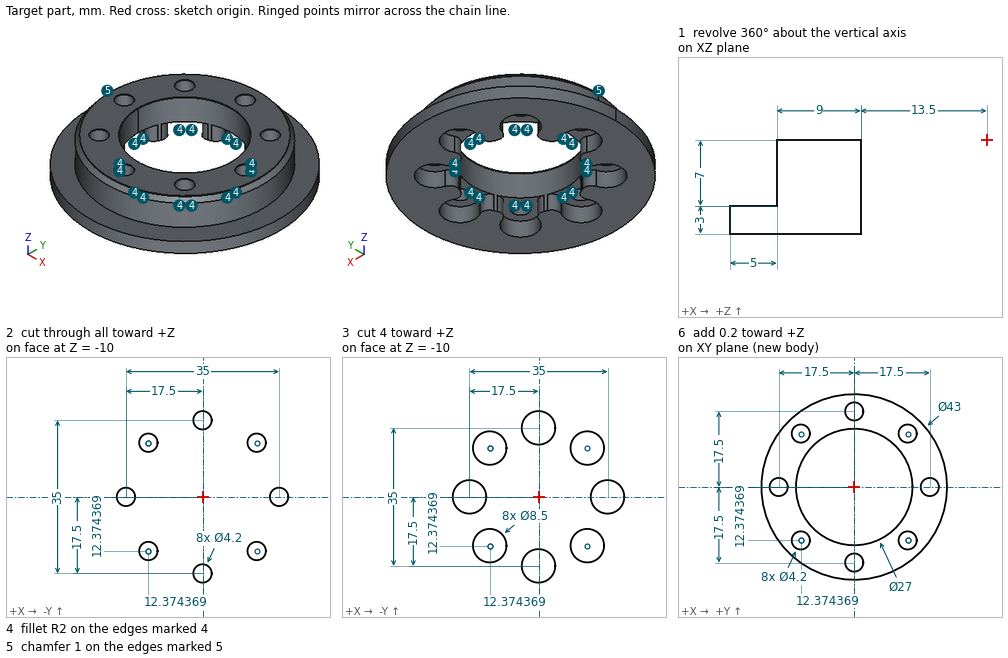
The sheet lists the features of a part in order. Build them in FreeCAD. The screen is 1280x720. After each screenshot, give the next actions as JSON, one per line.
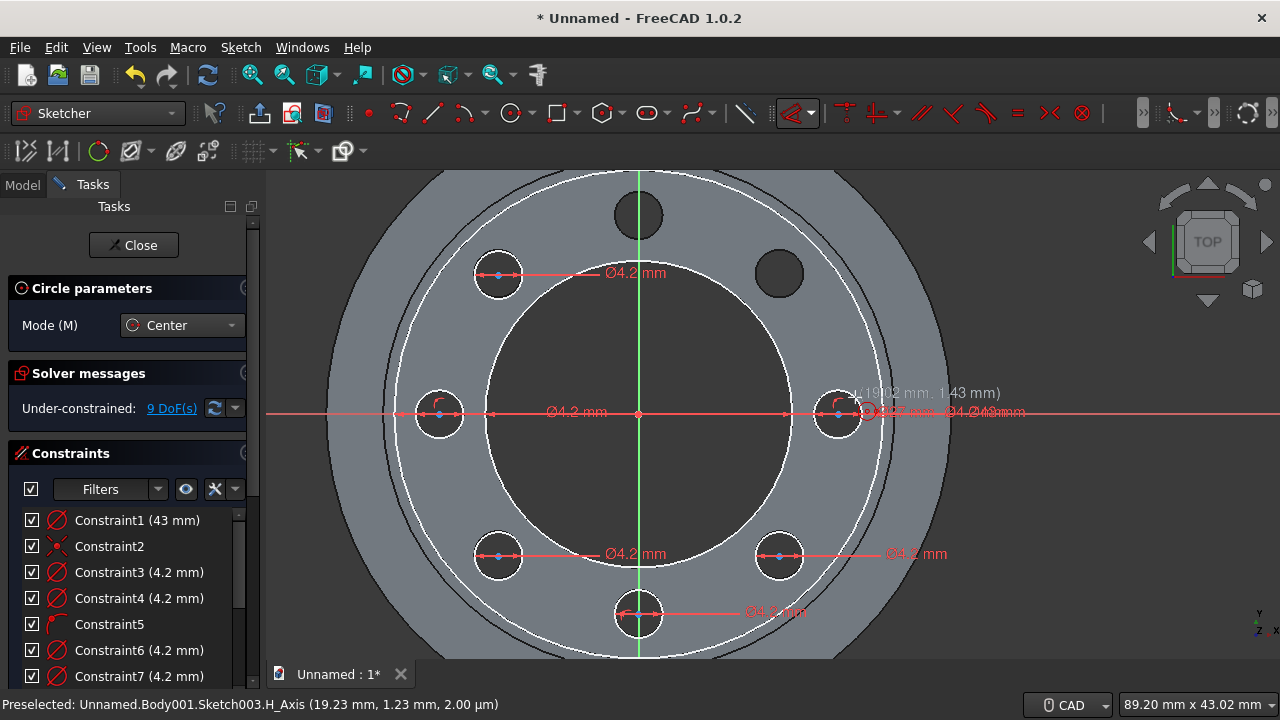
{"action": "left_click", "coordinate": [639, 215]}
{"action": "mouse_move", "coordinate": [656, 198]}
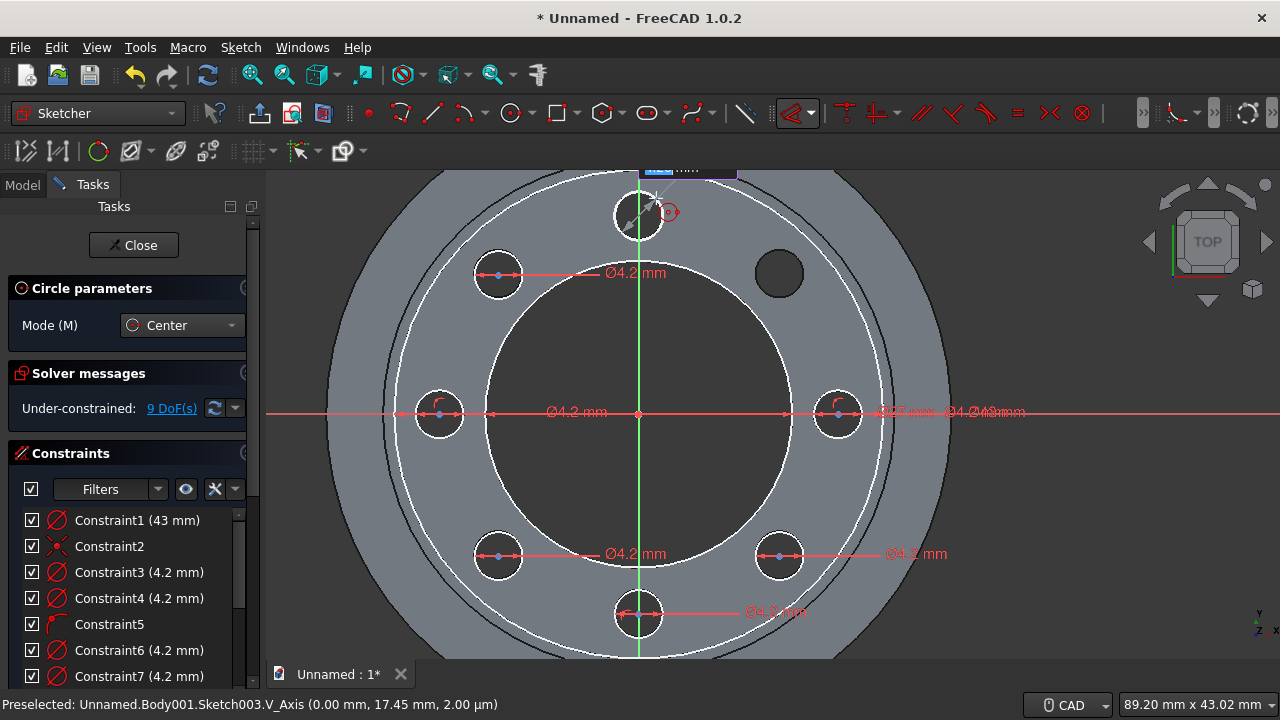
{"action": "type", "text": "4.2"}
{"action": "key", "text": "Return"}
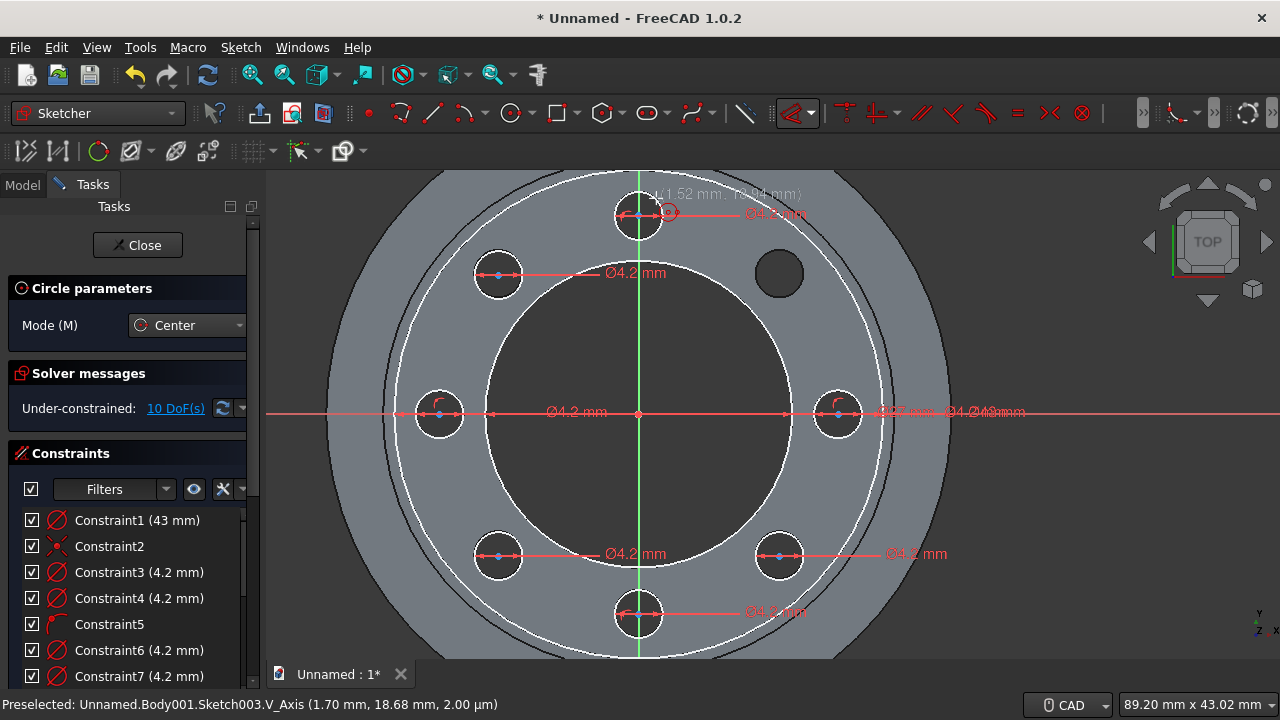
{"action": "left_click", "coordinate": [779, 274]}
{"action": "mouse_move", "coordinate": [796, 257]}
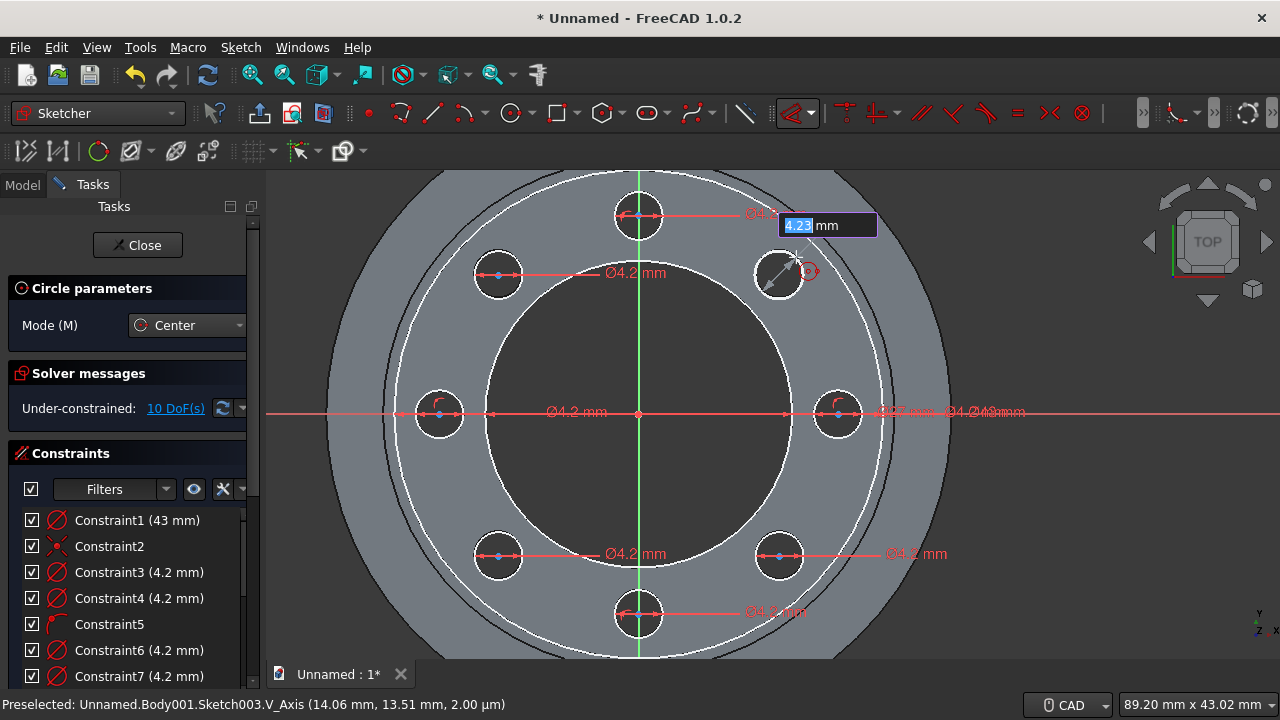
{"action": "type", "text": "4.2"}
{"action": "key", "text": "Return"}
{"action": "key", "text": "Escape"}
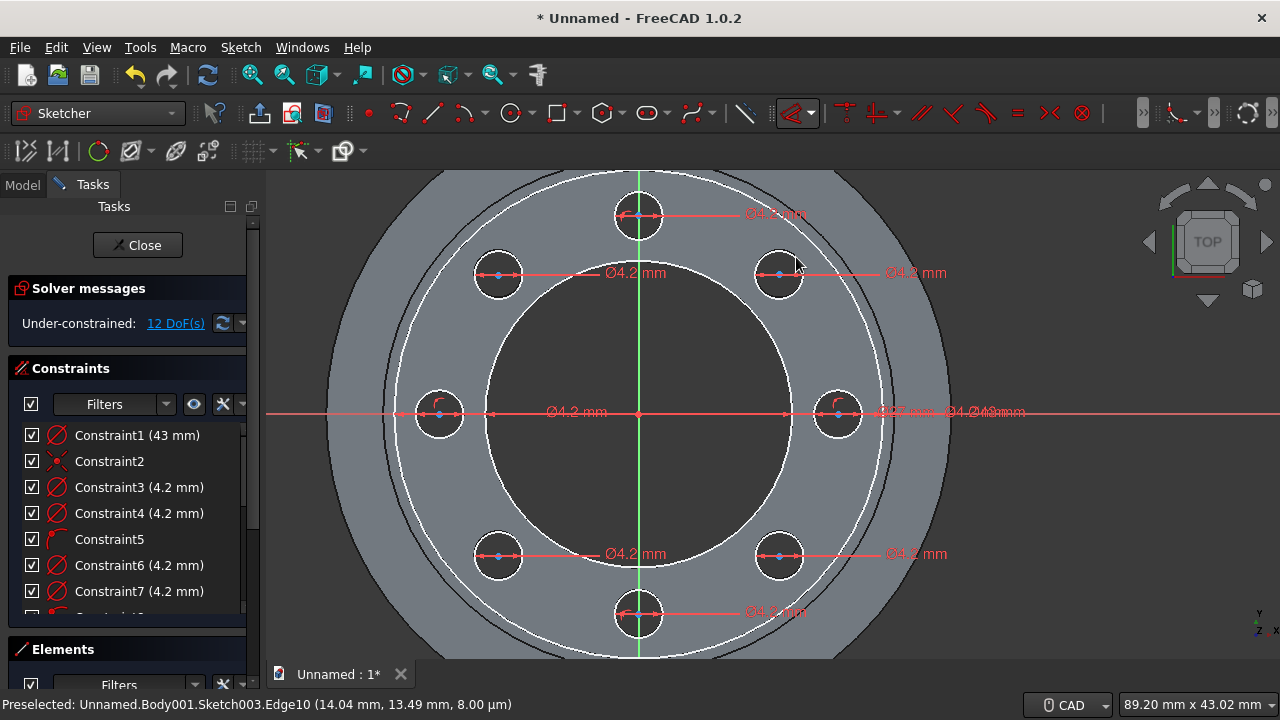
{"action": "left_click", "coordinate": [499, 556]}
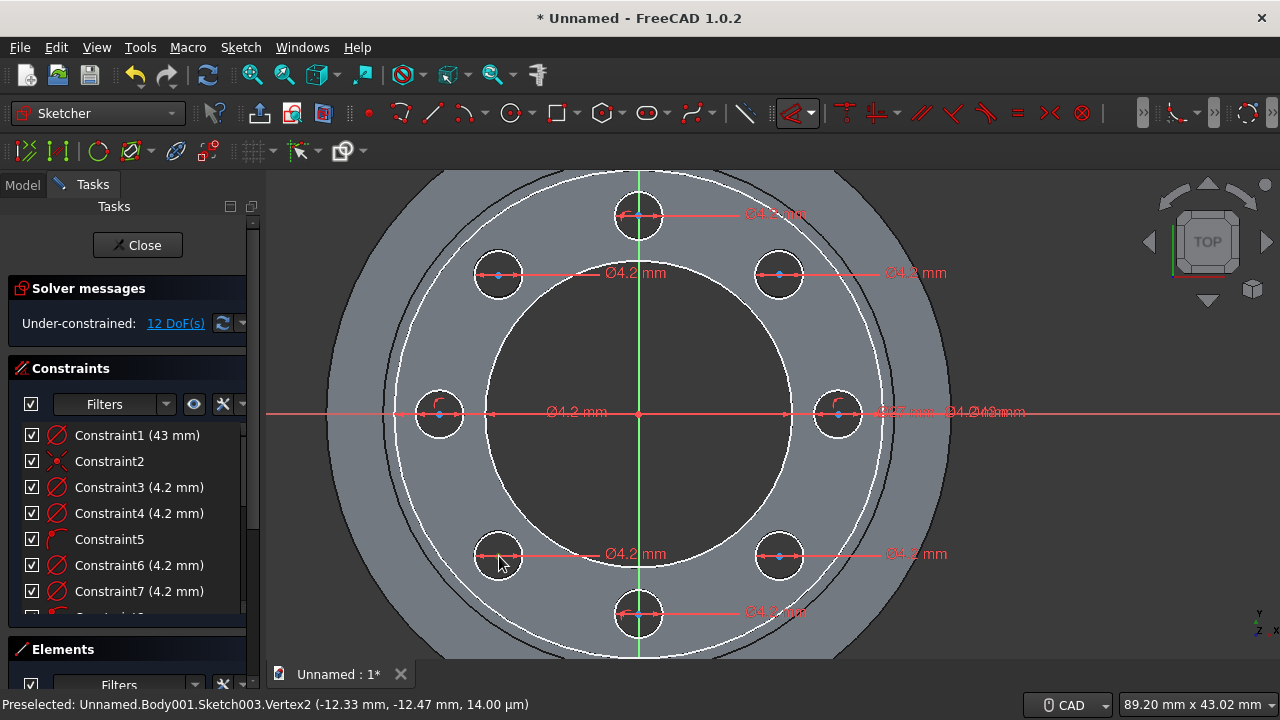
{"action": "left_click", "coordinate": [780, 556]}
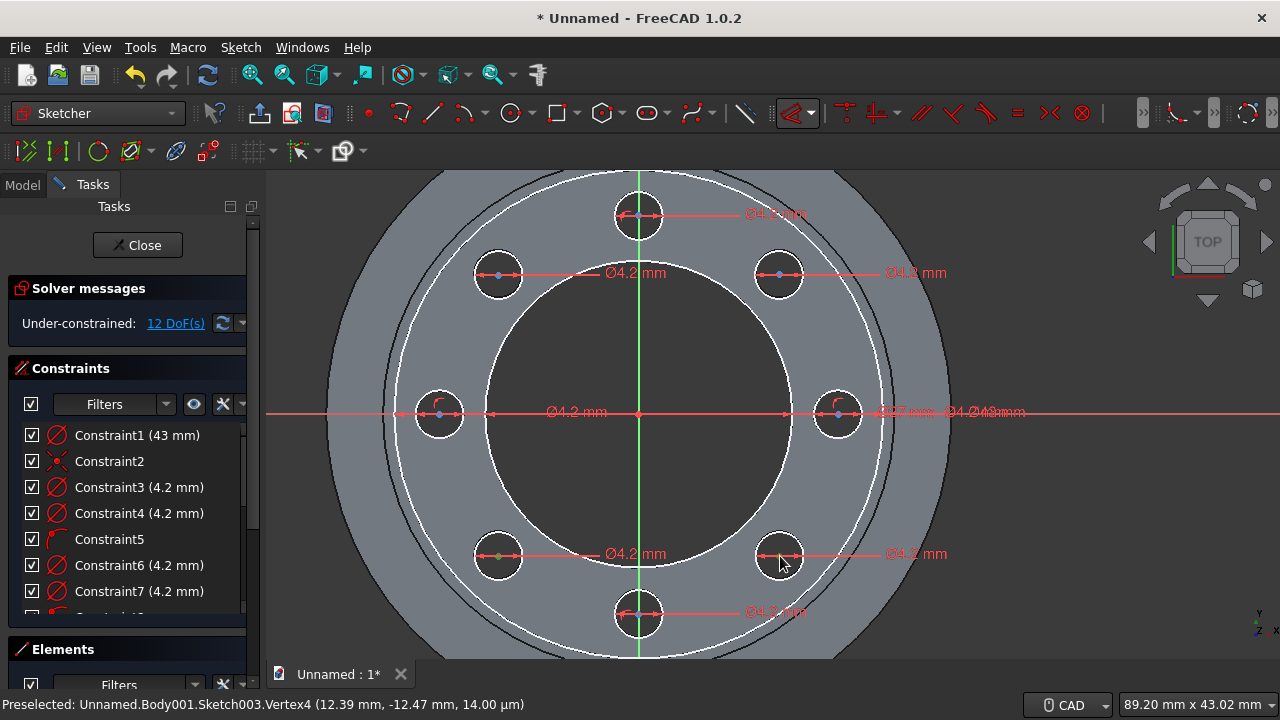
{"action": "left_click", "coordinate": [639, 507]}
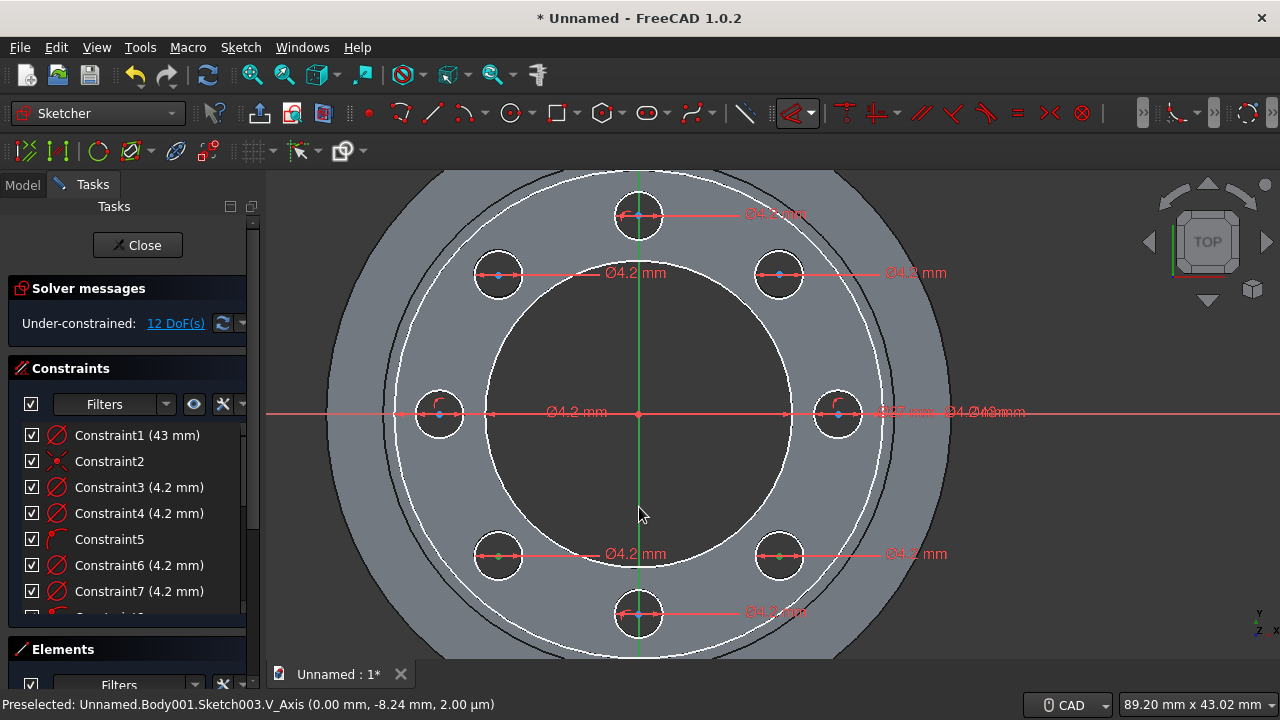
{"action": "left_click", "coordinate": [1050, 114]}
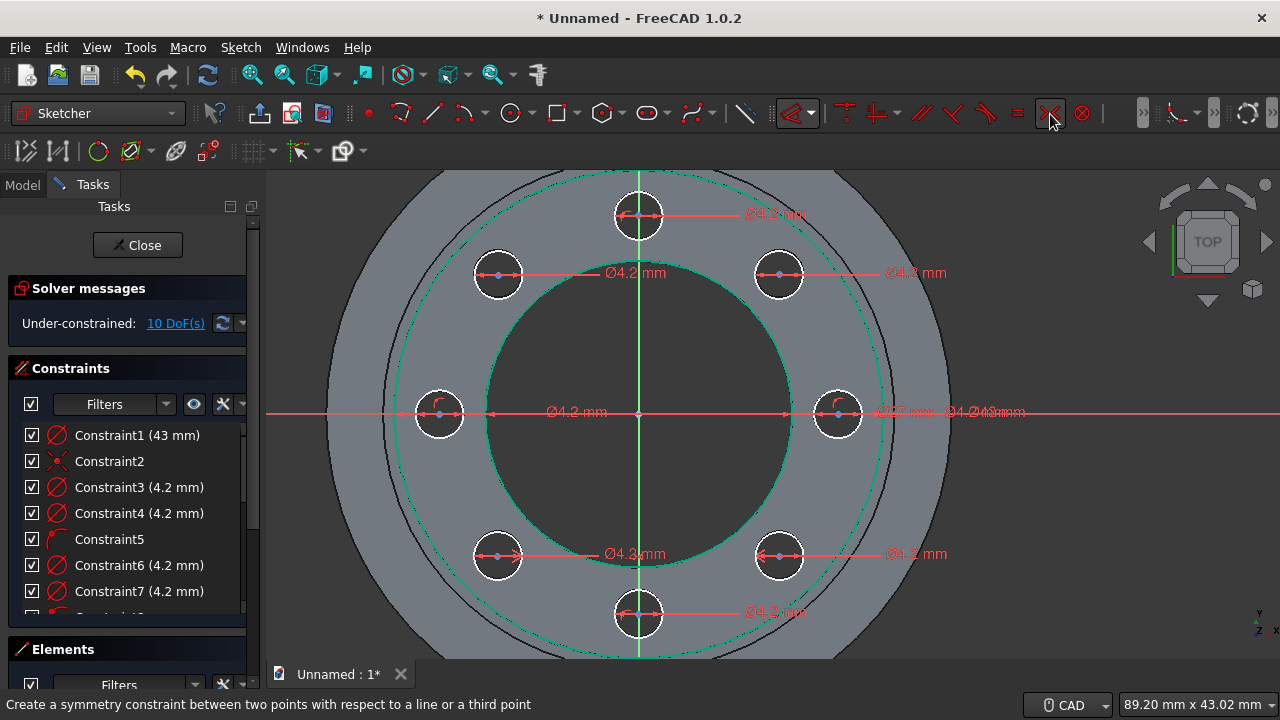
{"action": "left_click", "coordinate": [498, 556]}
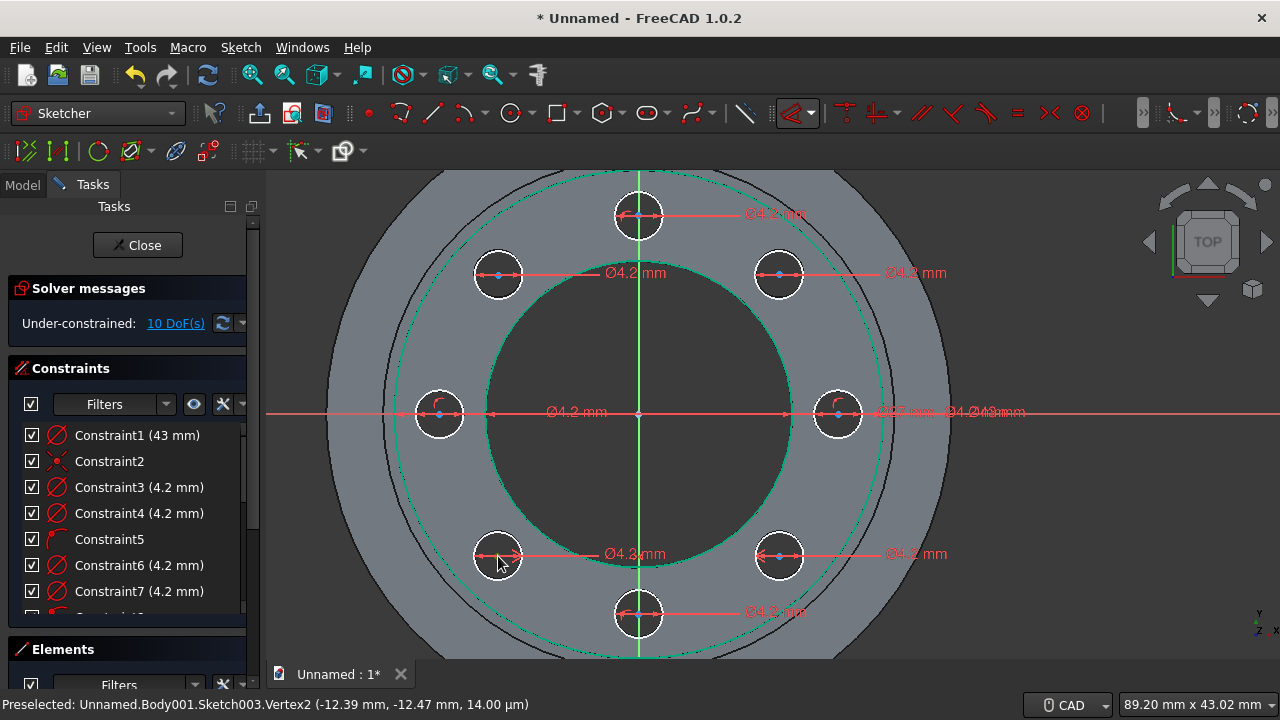
{"action": "left_click", "coordinate": [499, 275]}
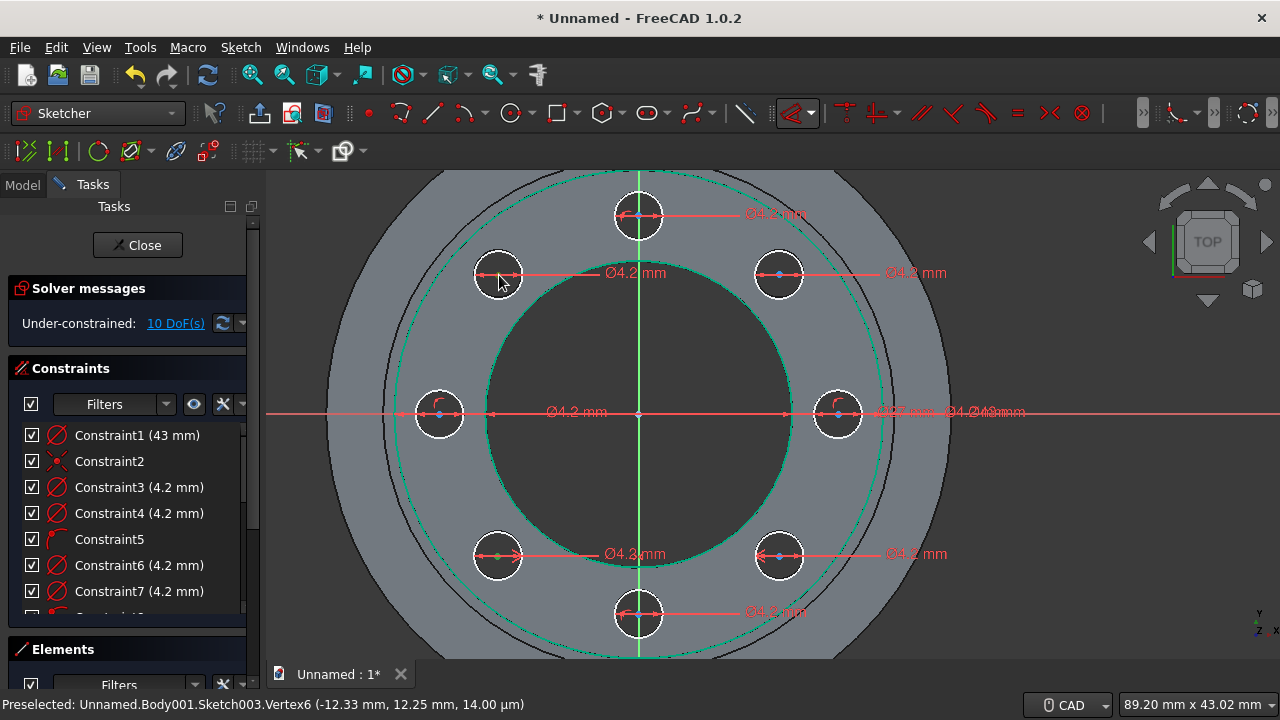
{"action": "left_click", "coordinate": [353, 414]}